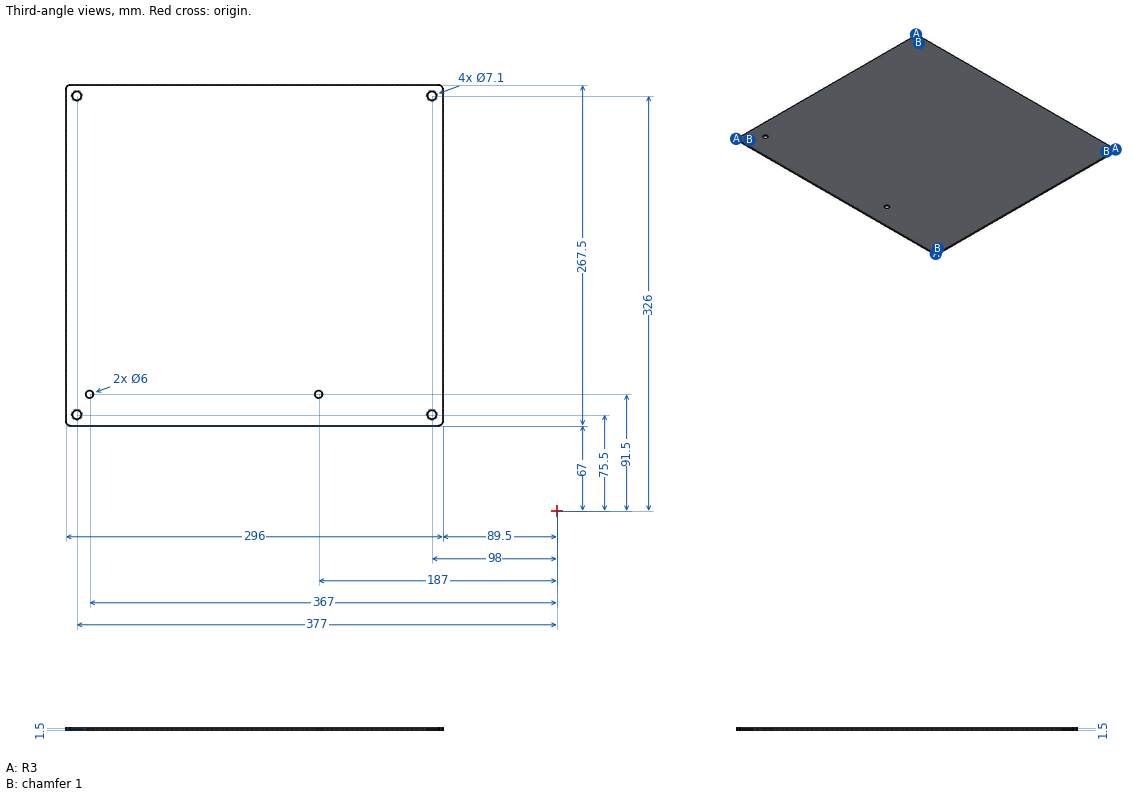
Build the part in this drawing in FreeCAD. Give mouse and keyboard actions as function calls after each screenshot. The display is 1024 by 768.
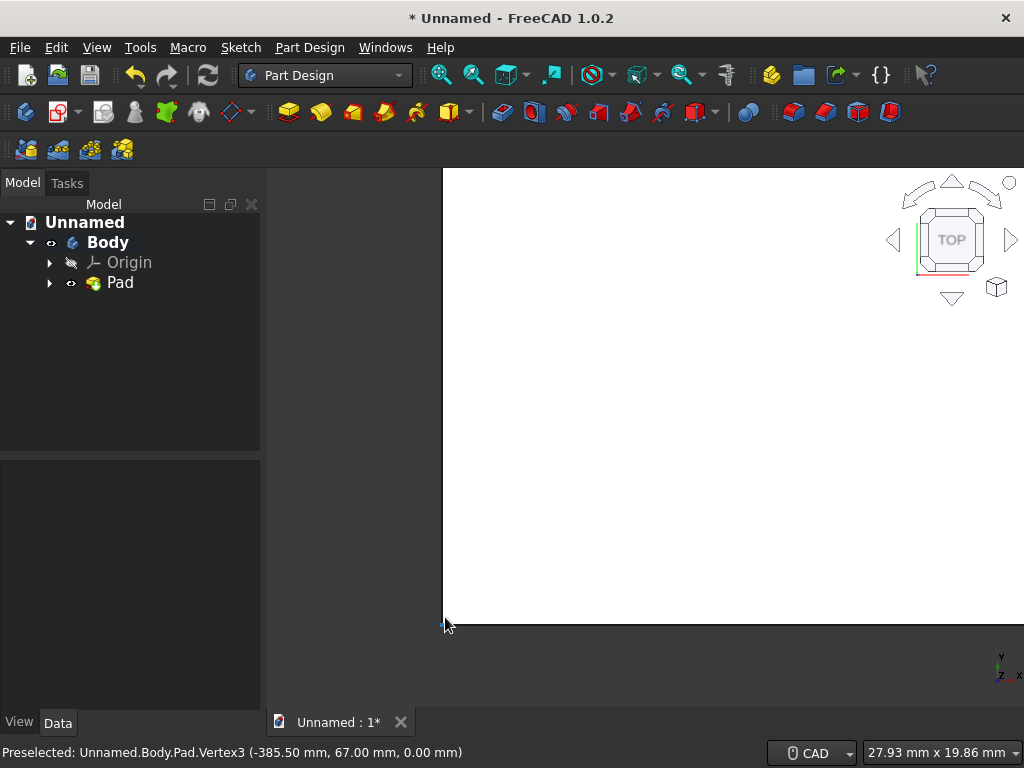
click(442, 76)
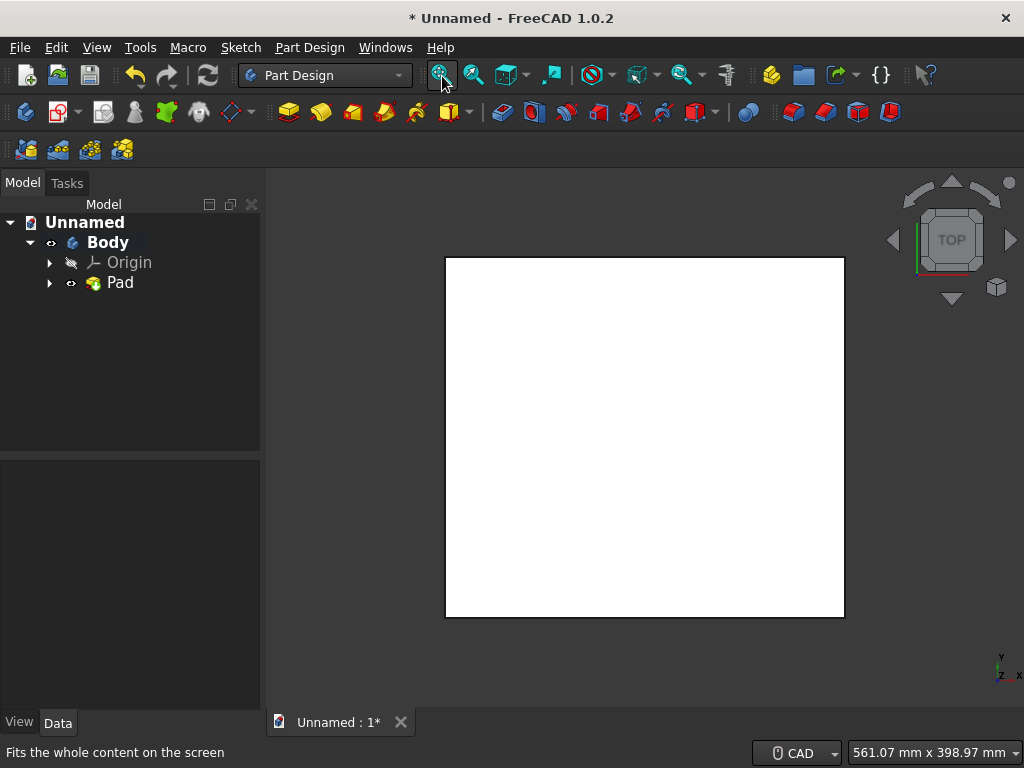
key(1)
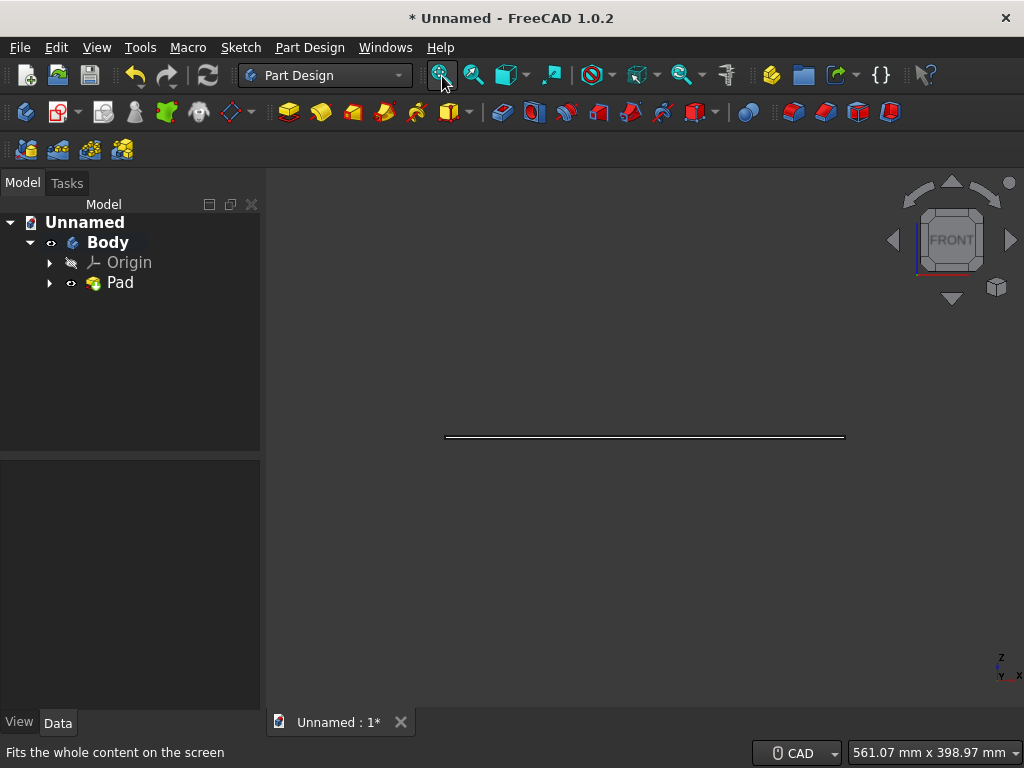
scroll(445, 436, up, 15)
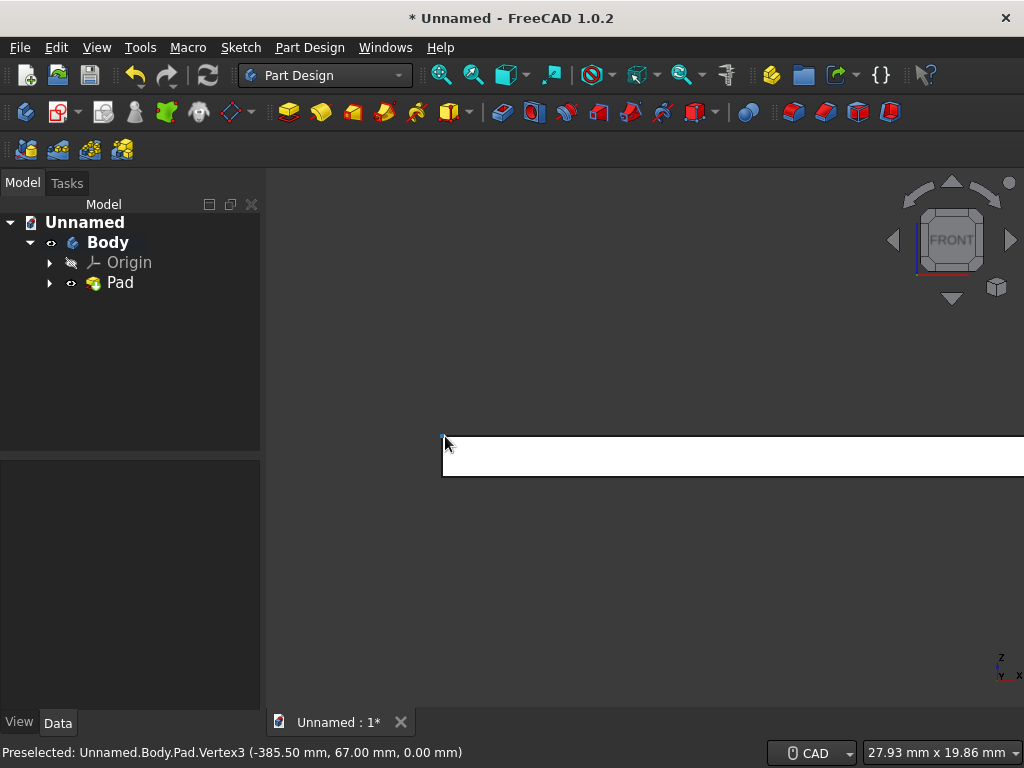
click(442, 456)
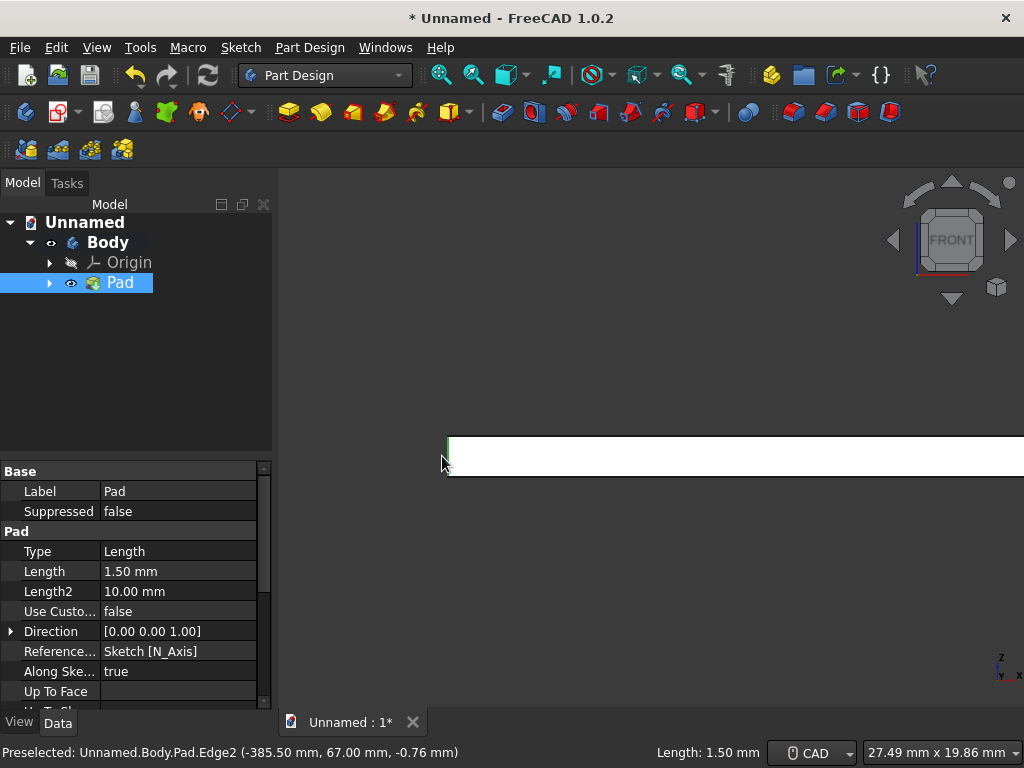
click(442, 76)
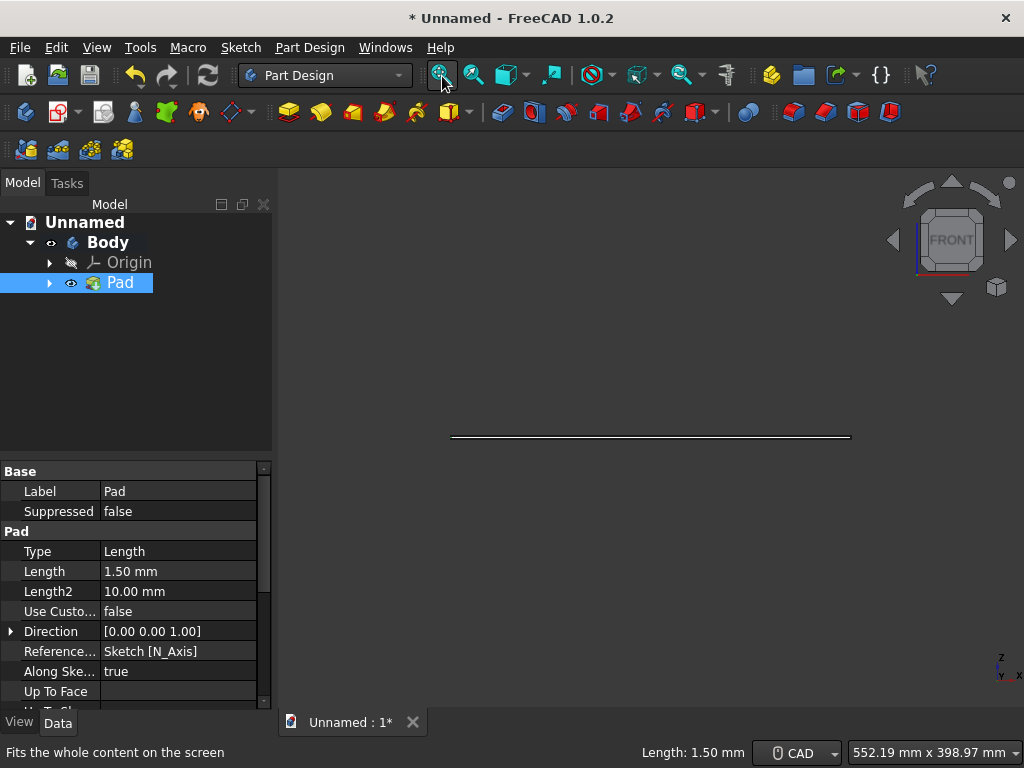
key(3)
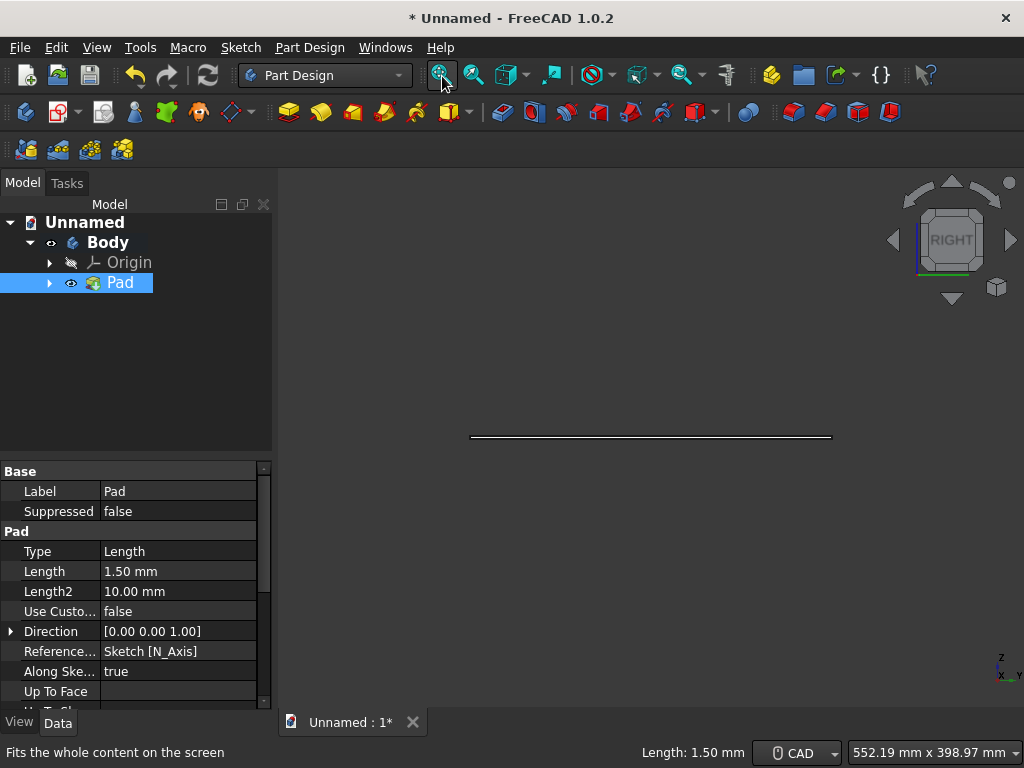
scroll(832, 436, up, 15)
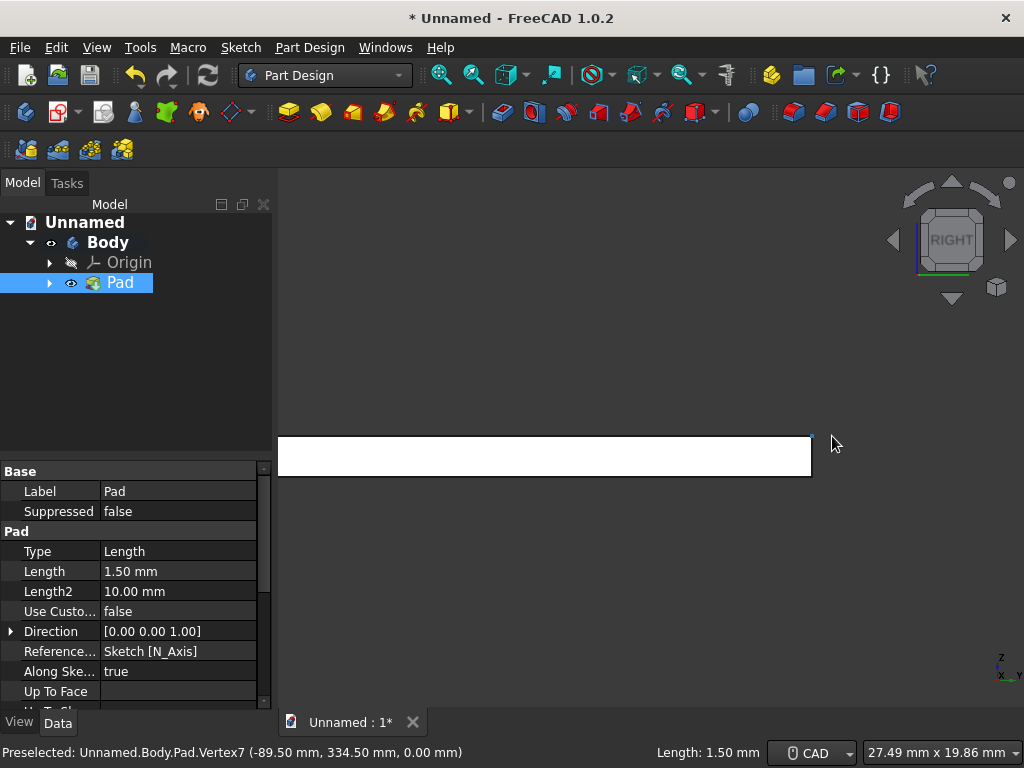
click(812, 456, ctrl)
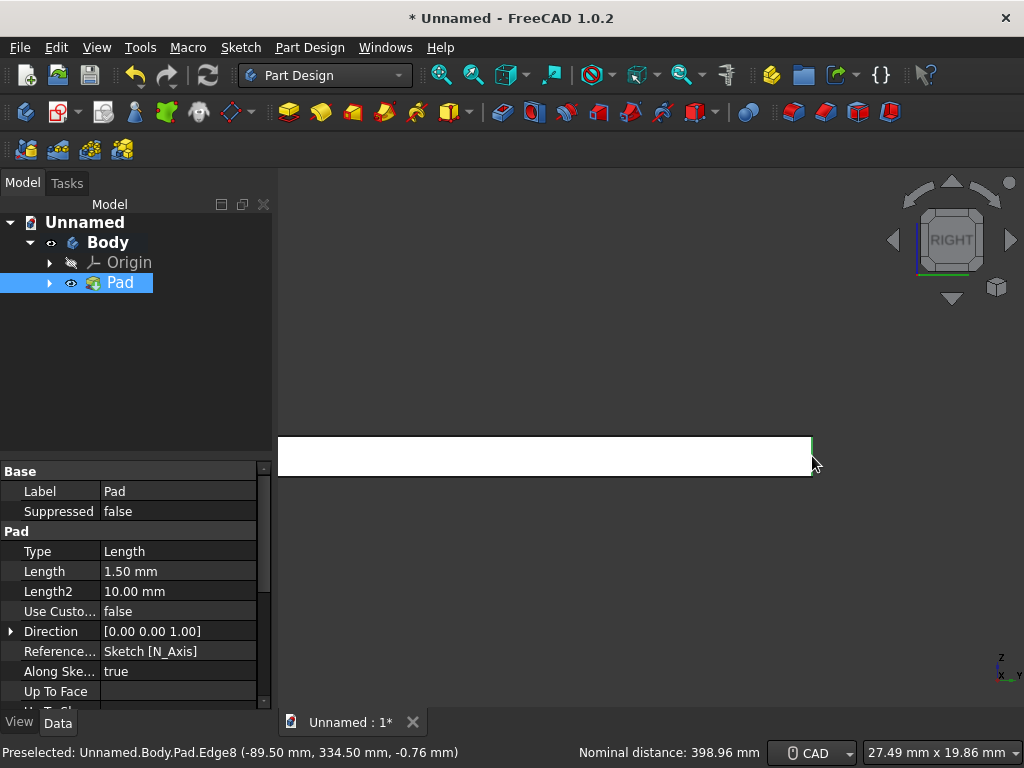
click(442, 76)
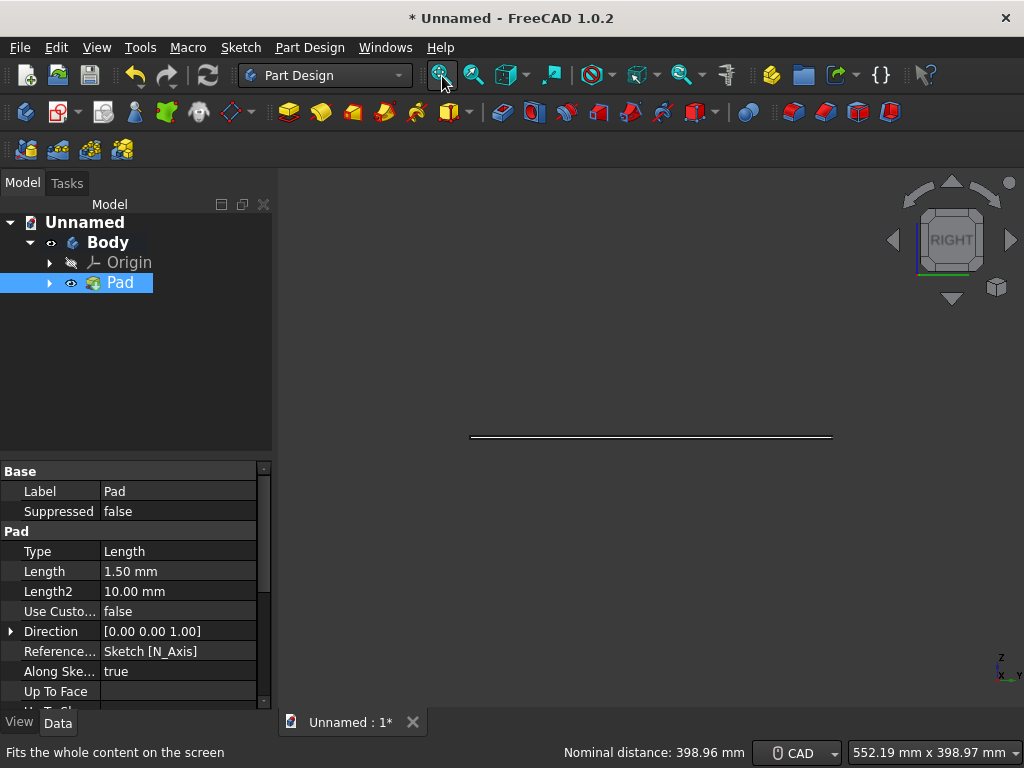
key(5)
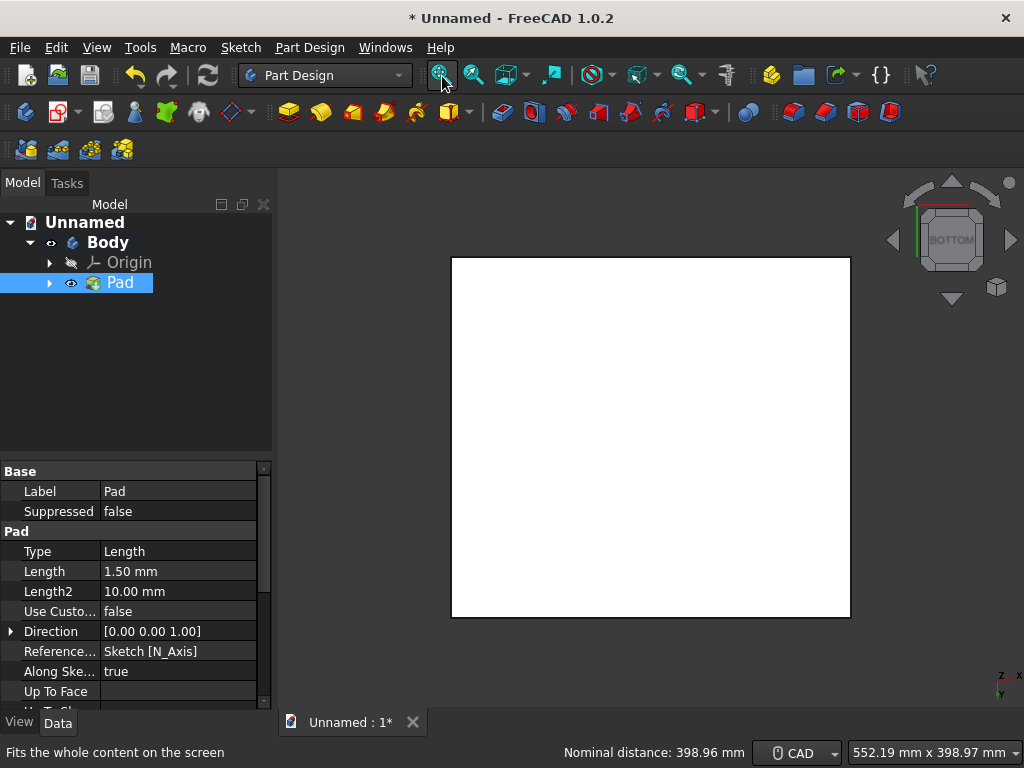
scroll(451, 617, up, 15)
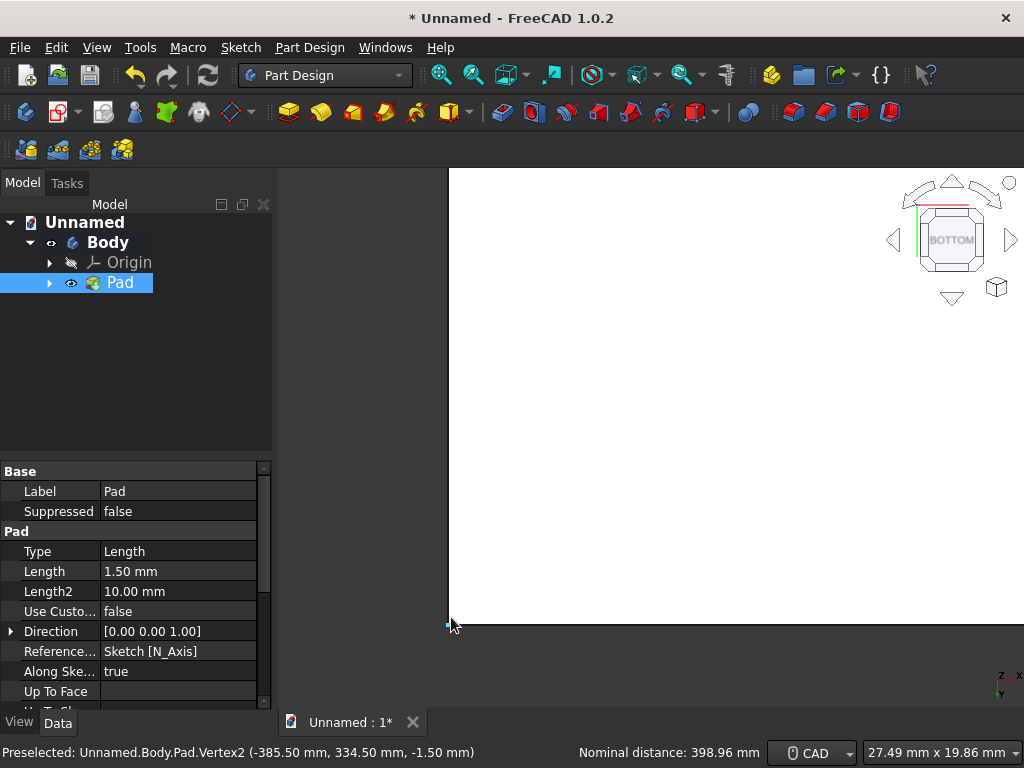
click(442, 76)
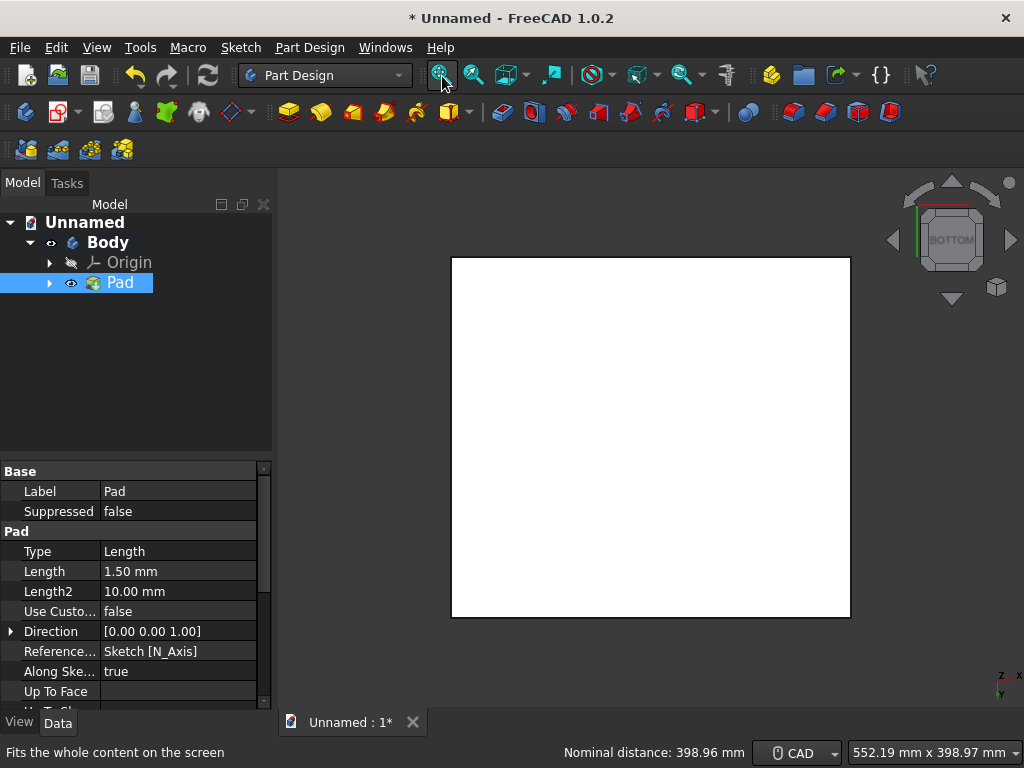
key(4)